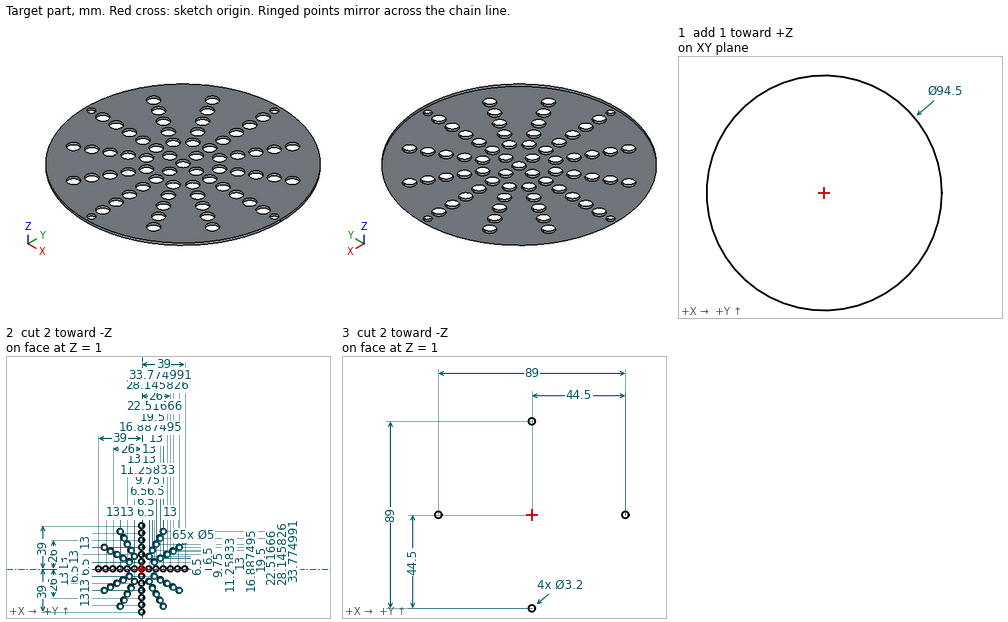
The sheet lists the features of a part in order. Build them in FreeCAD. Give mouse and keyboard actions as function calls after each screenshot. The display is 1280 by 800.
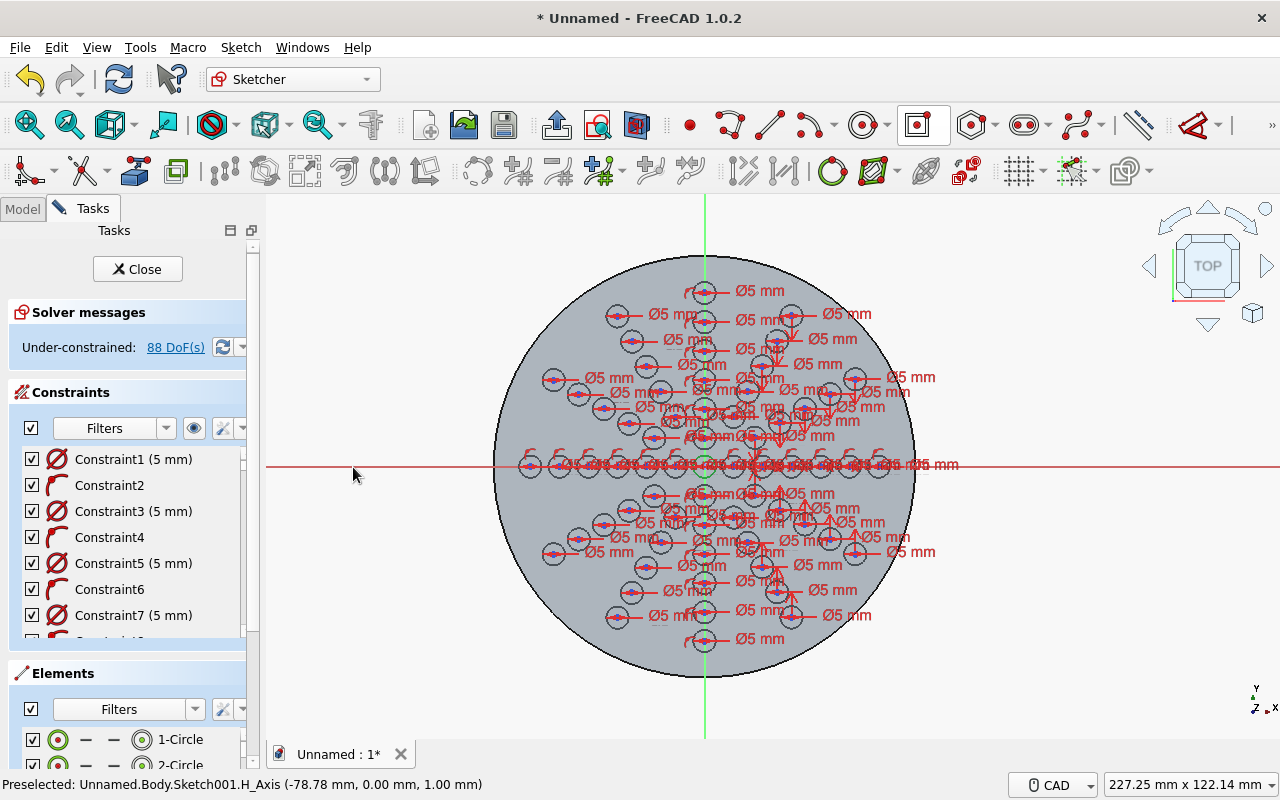
click(748, 392)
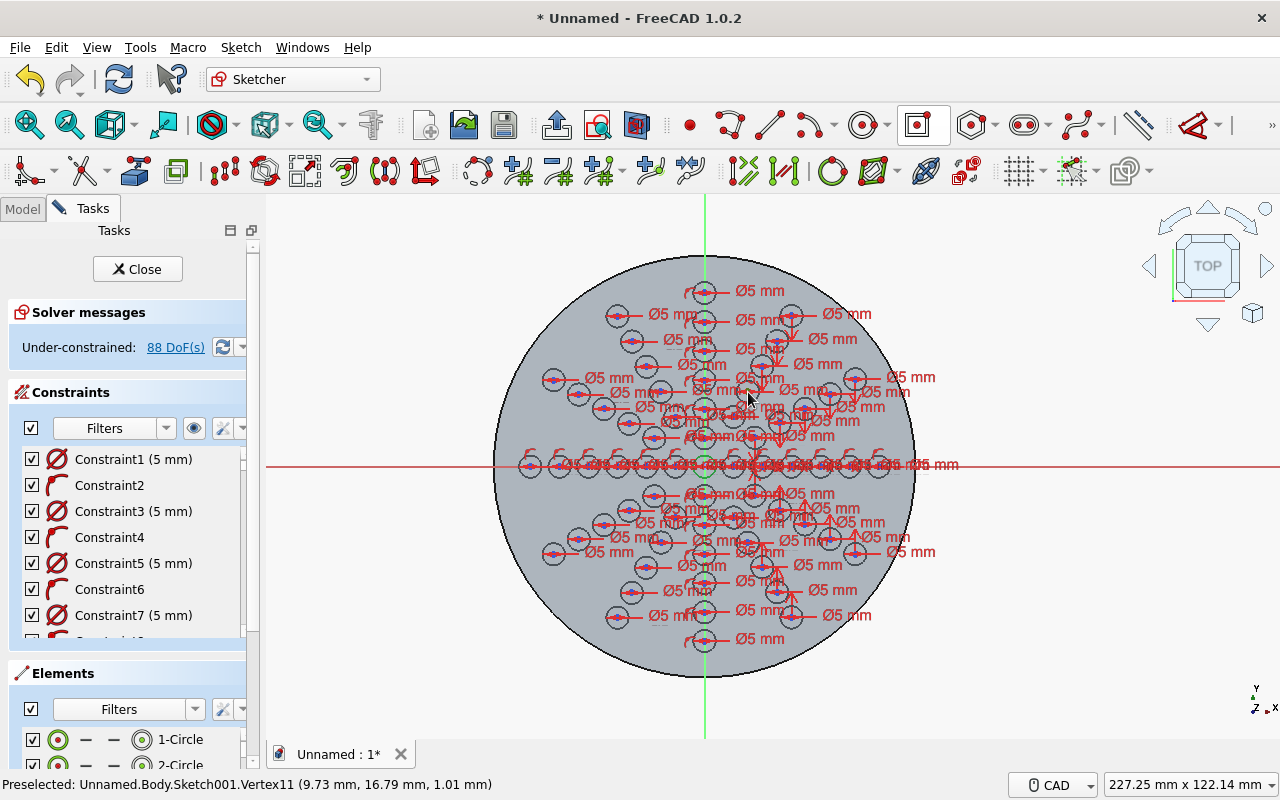
click(748, 543)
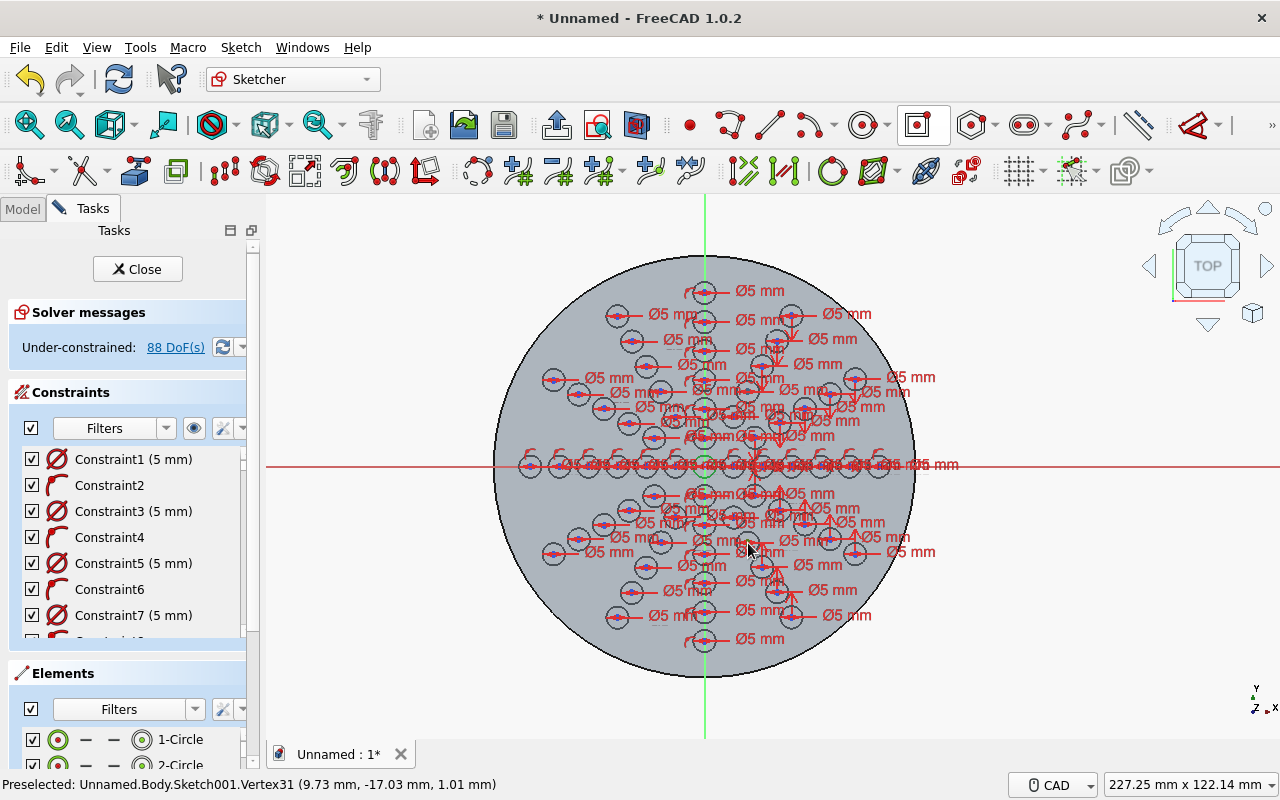
click(353, 467)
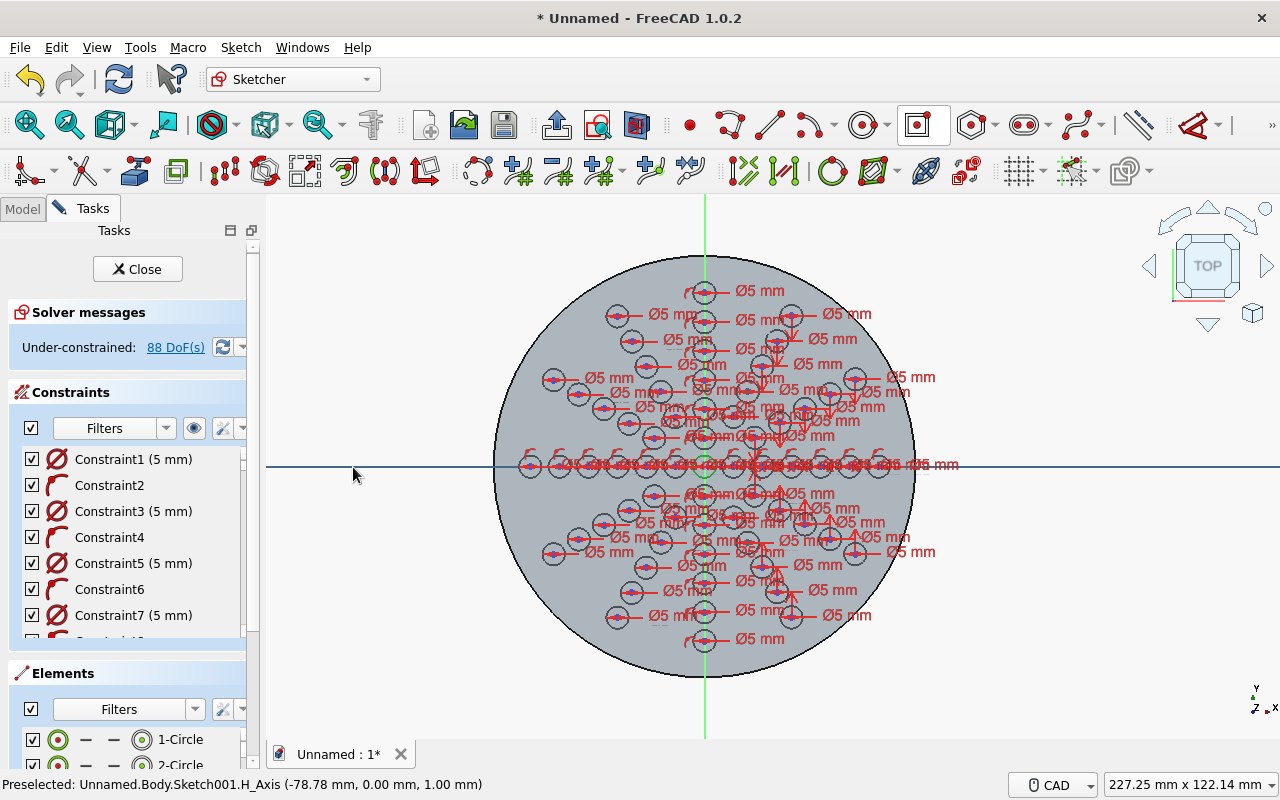
key(s)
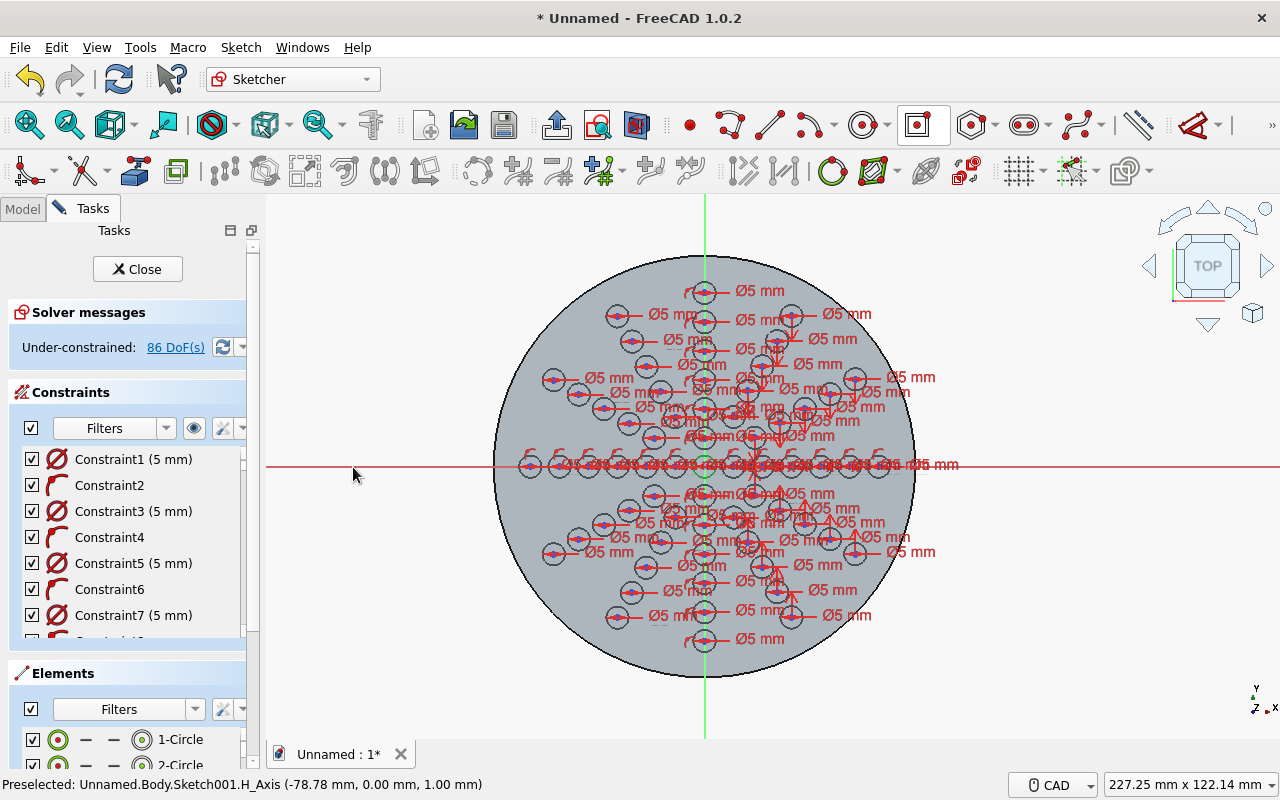
click(734, 417)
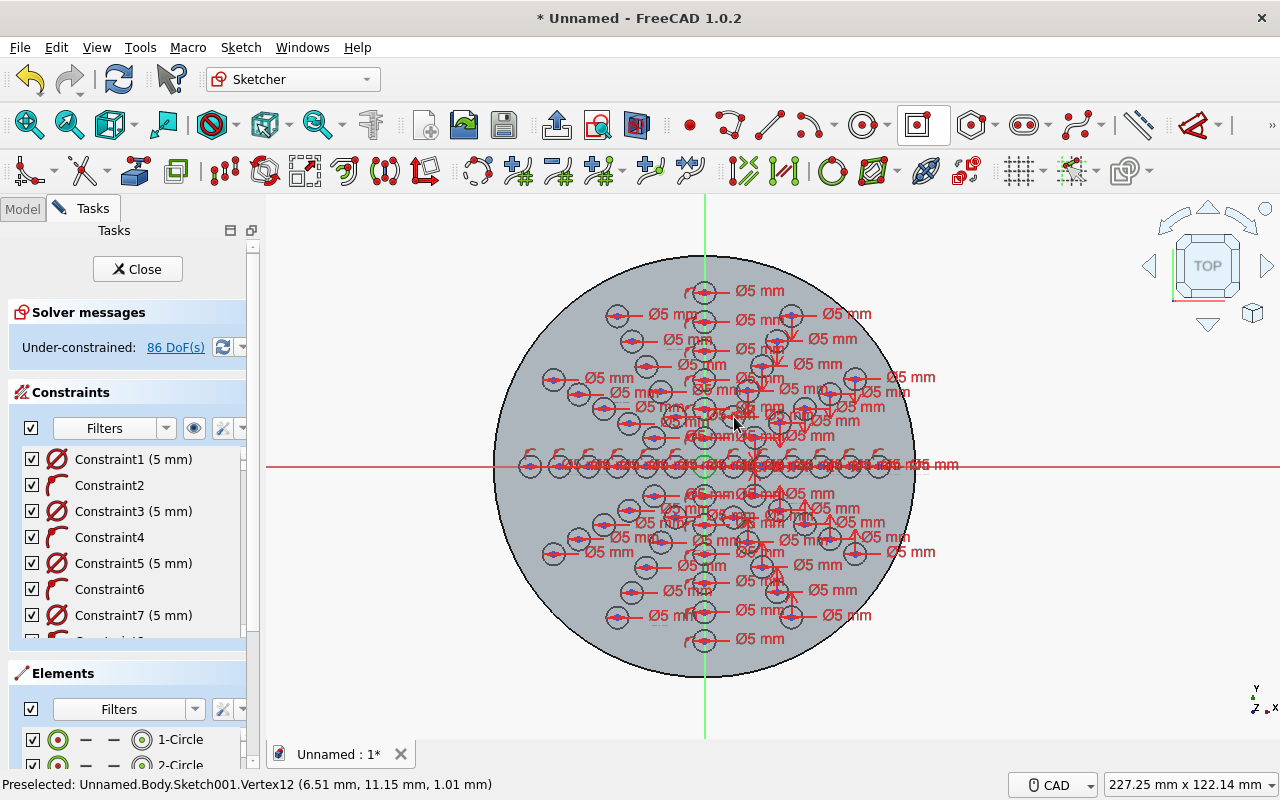
click(734, 518)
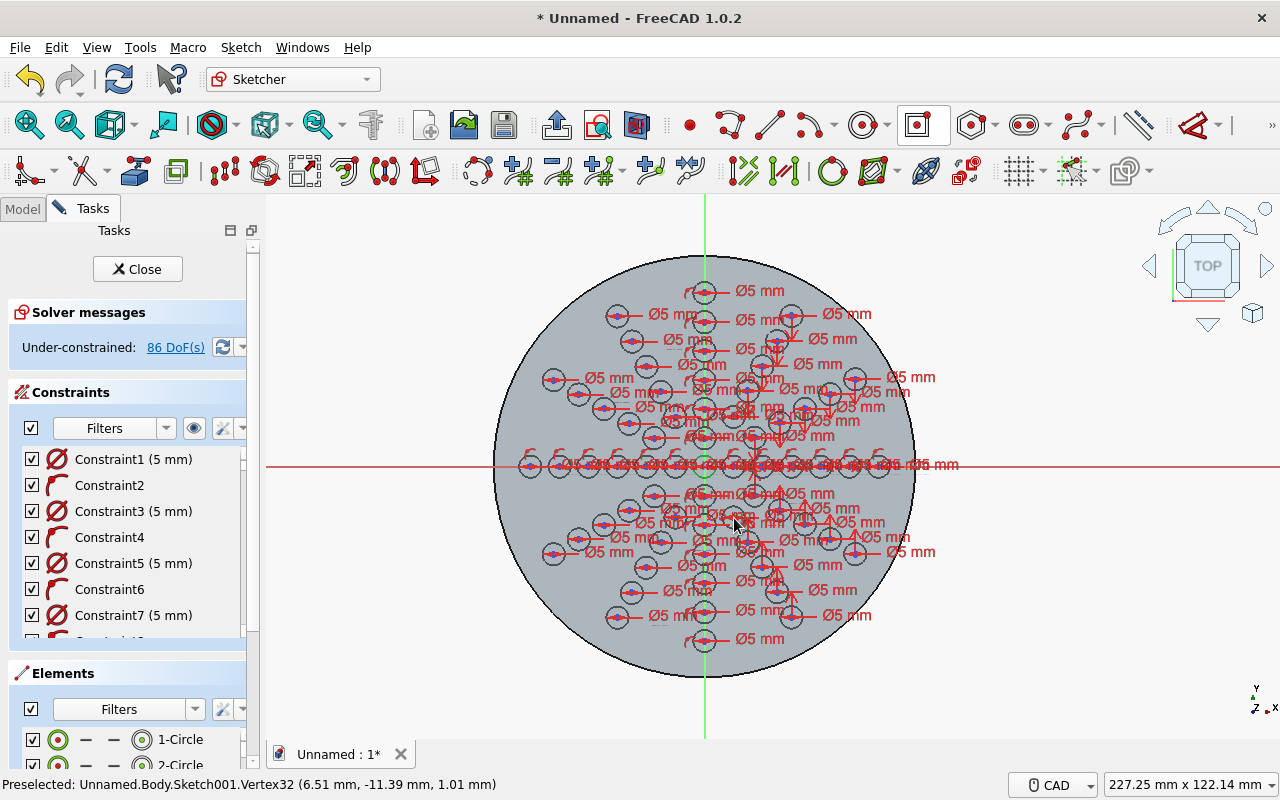
click(353, 467)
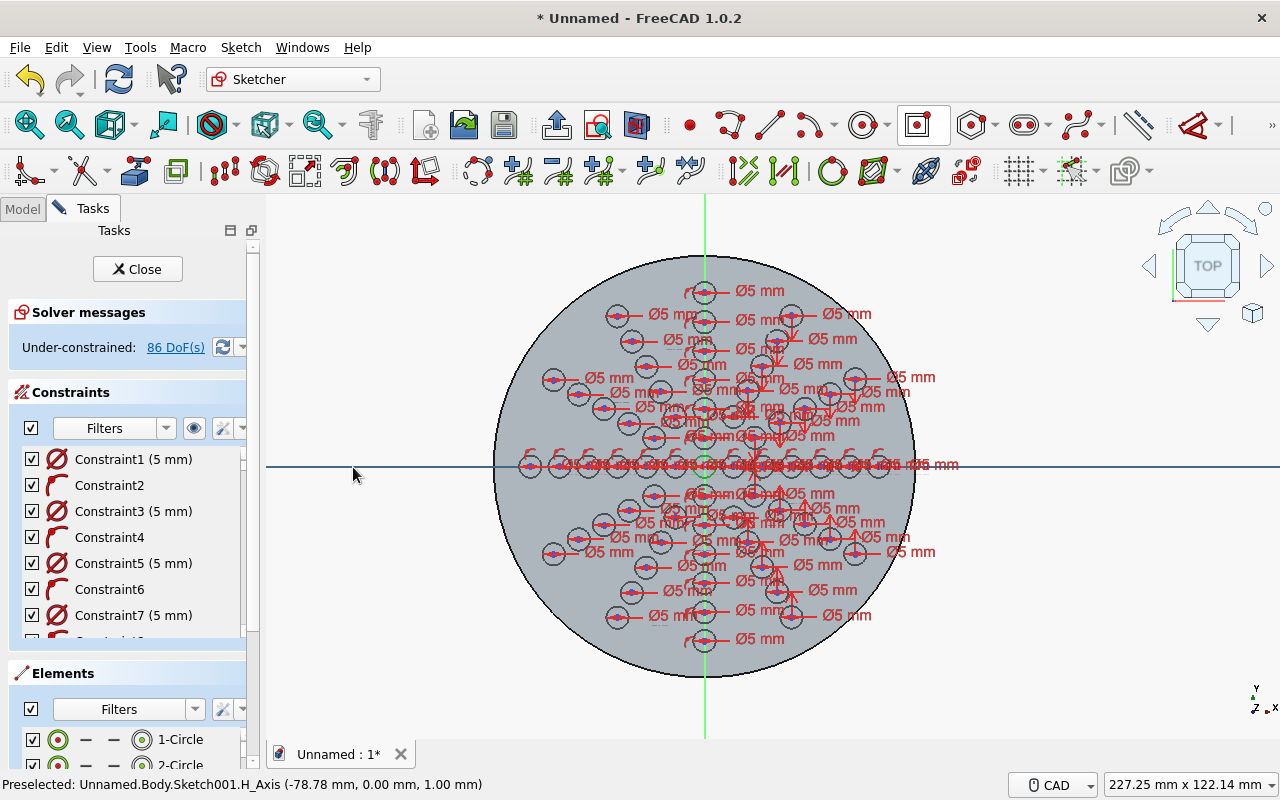
key(s)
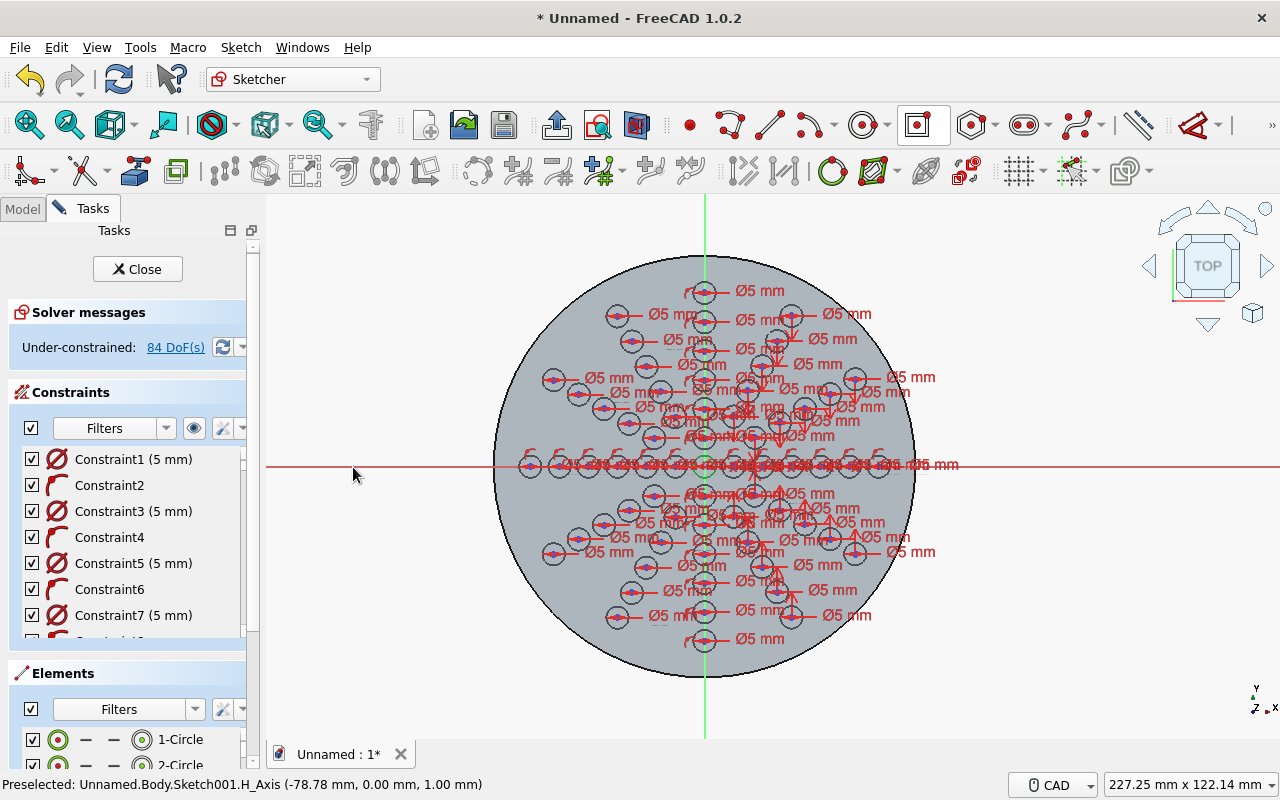
click(792, 617)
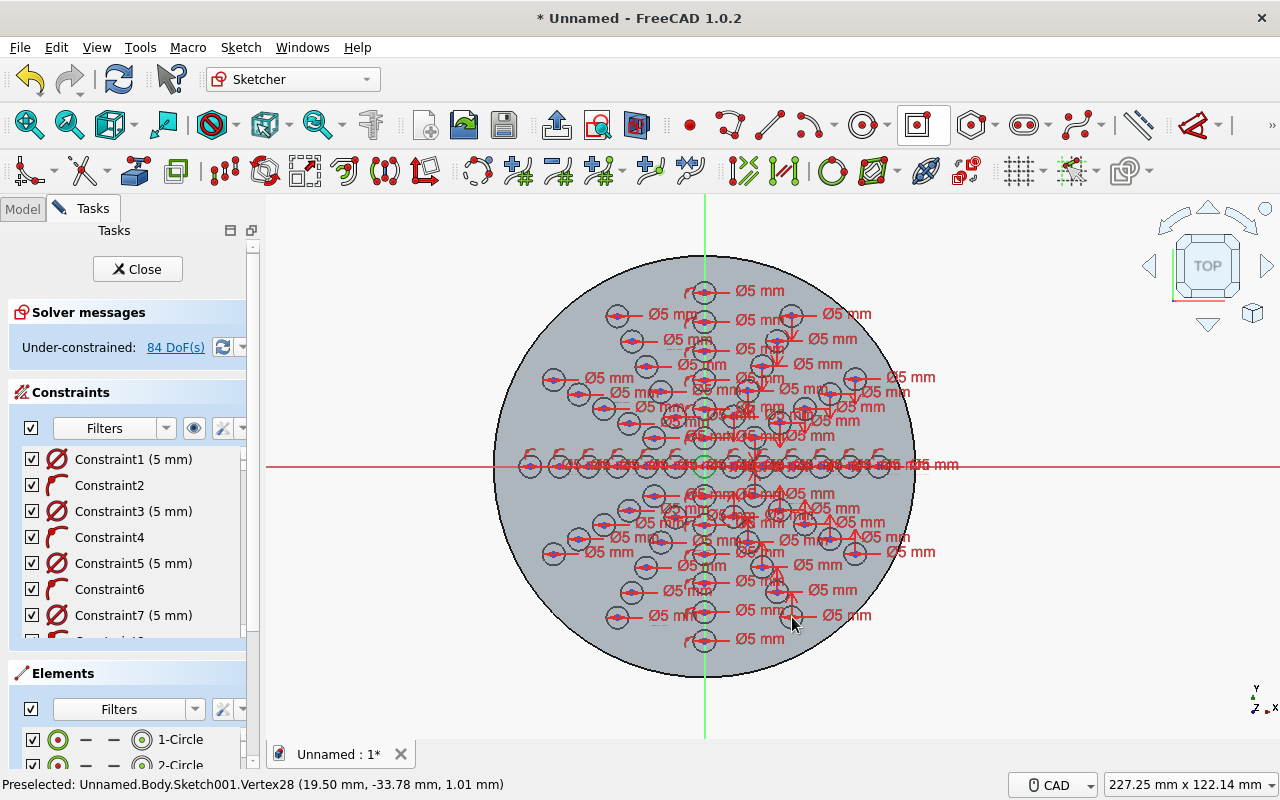
click(618, 618)